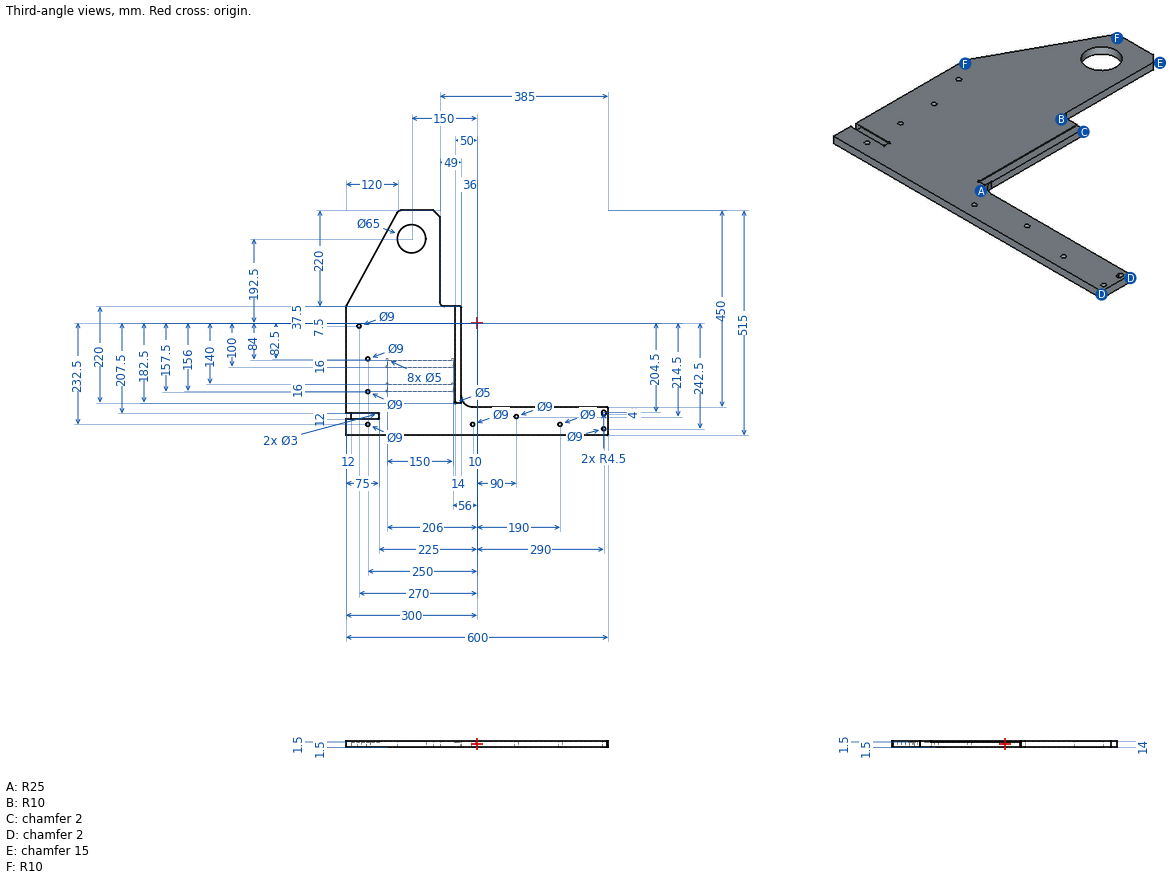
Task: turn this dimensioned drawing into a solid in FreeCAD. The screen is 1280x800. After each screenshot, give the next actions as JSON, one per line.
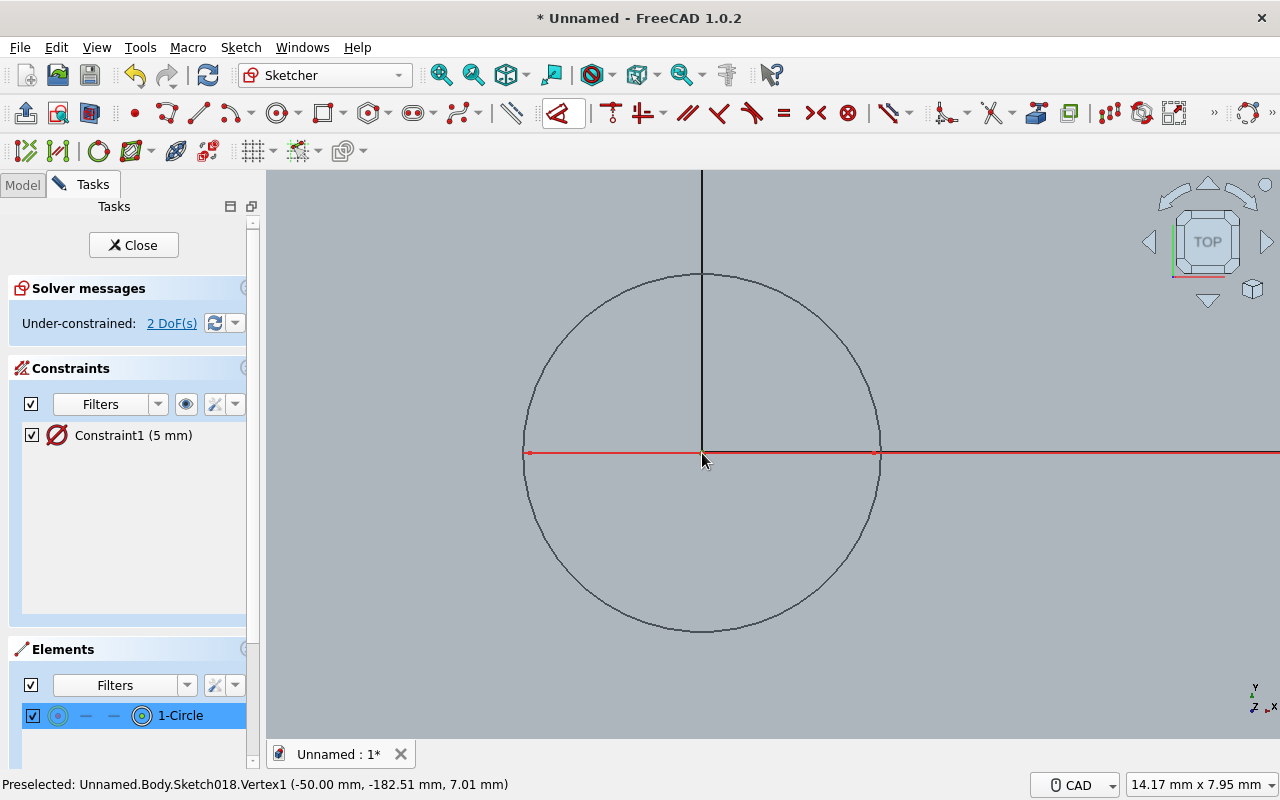
{"action": "left_click", "coordinate": [580, 114]}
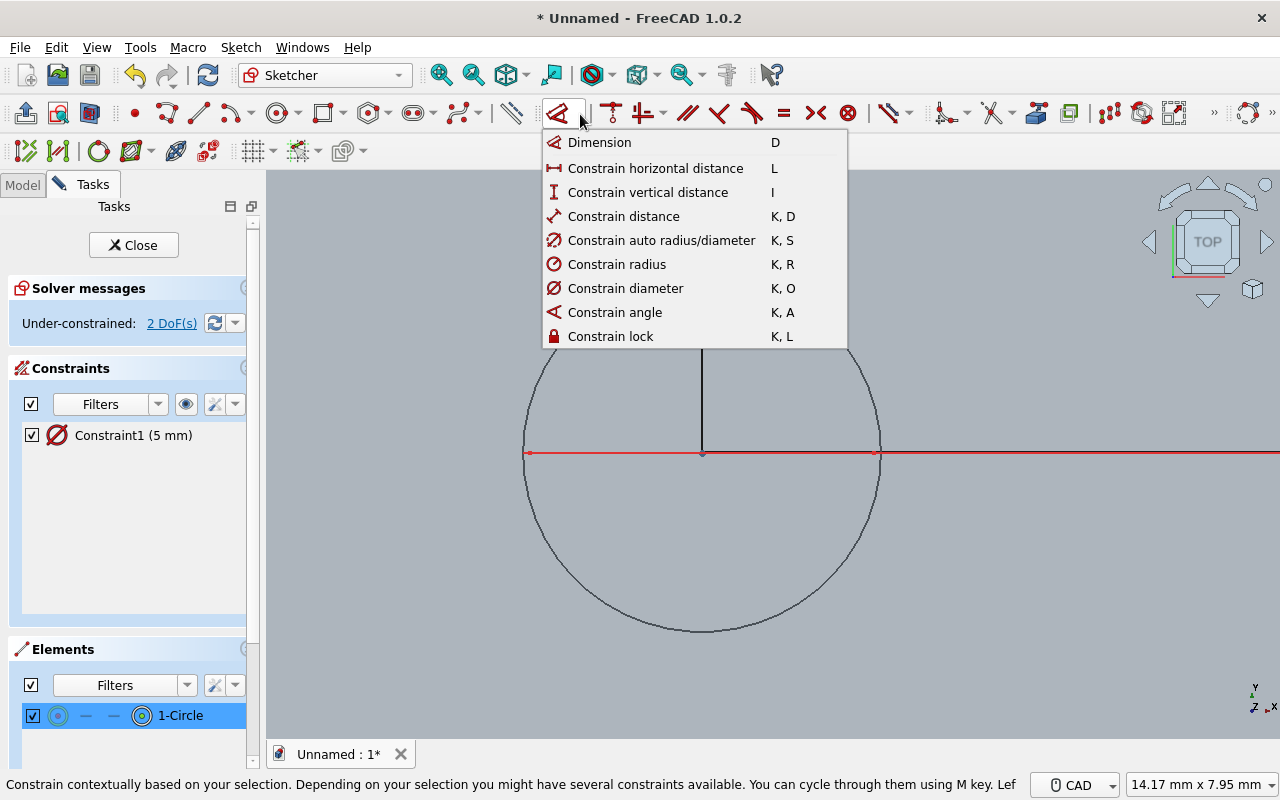
{"action": "left_click", "coordinate": [695, 168]}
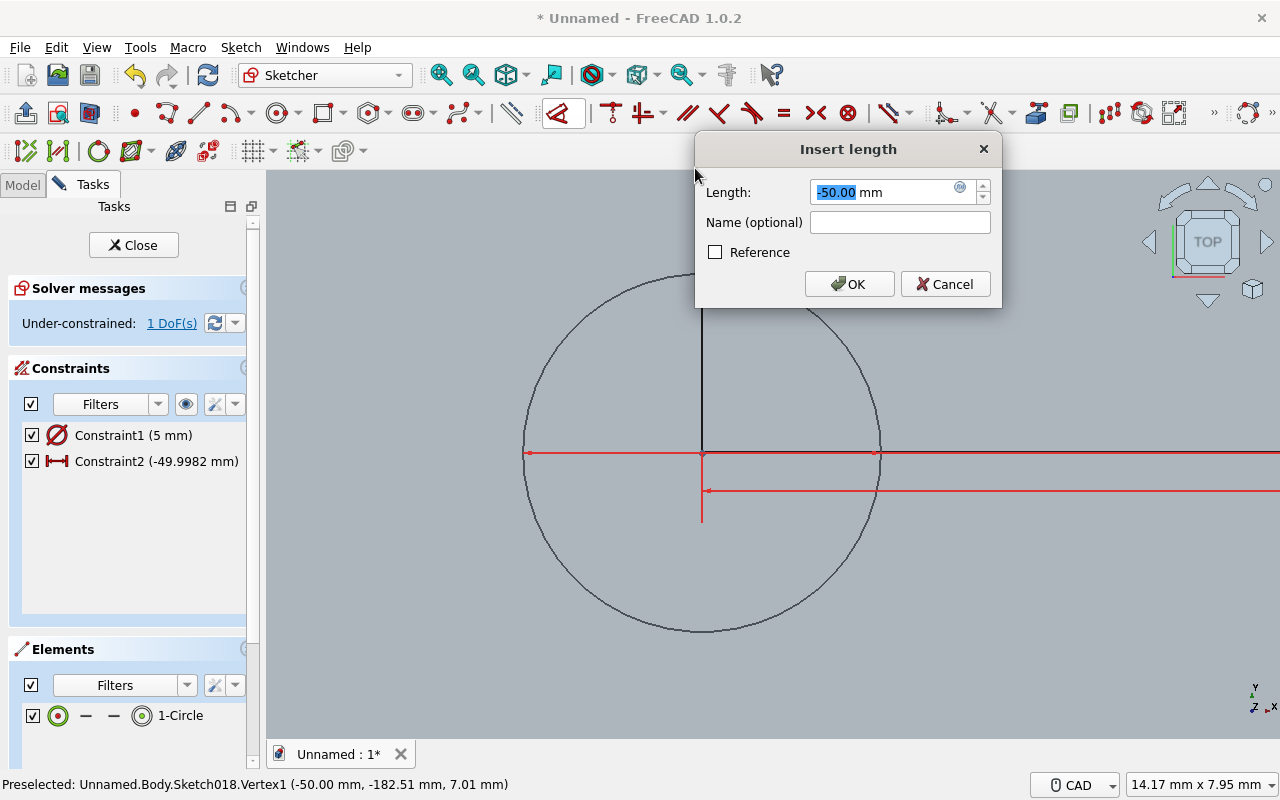
{"action": "type", "text": "-50"}
{"action": "key", "text": "Return"}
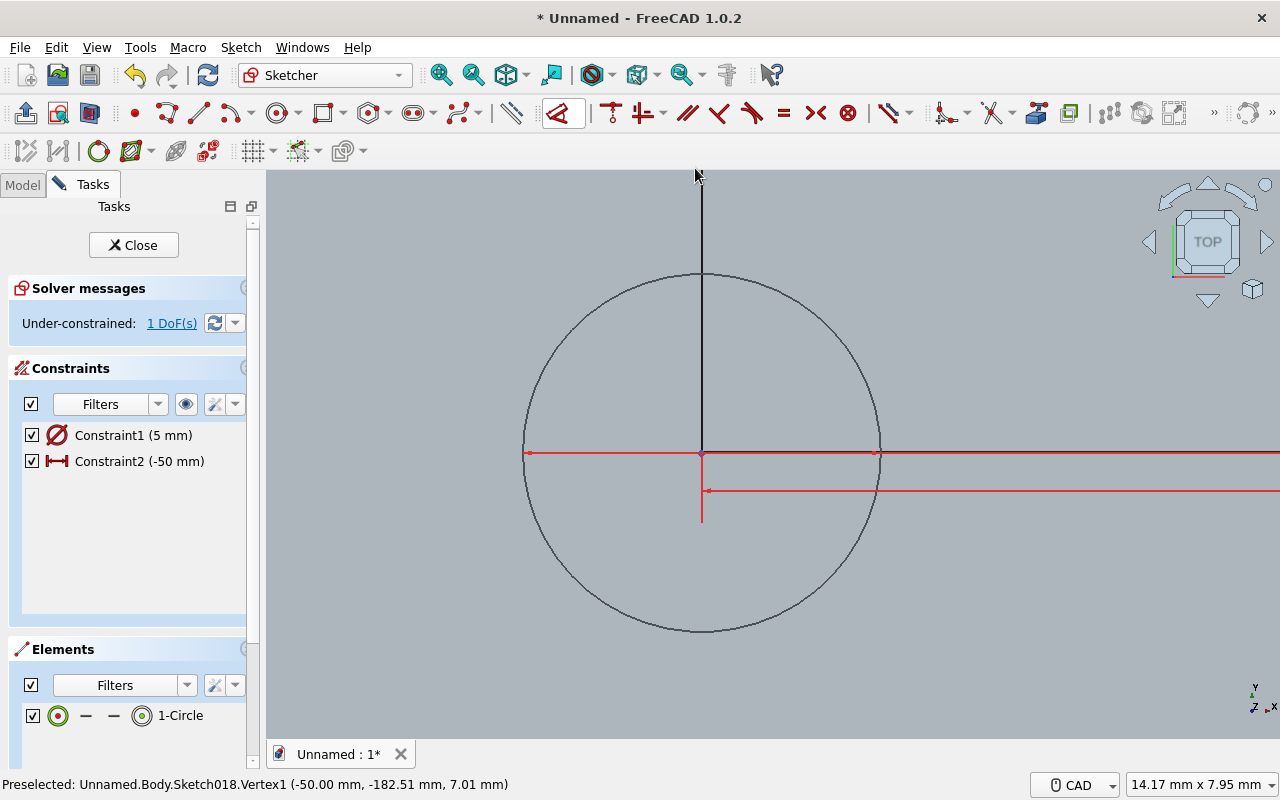
{"action": "left_click", "coordinate": [702, 453]}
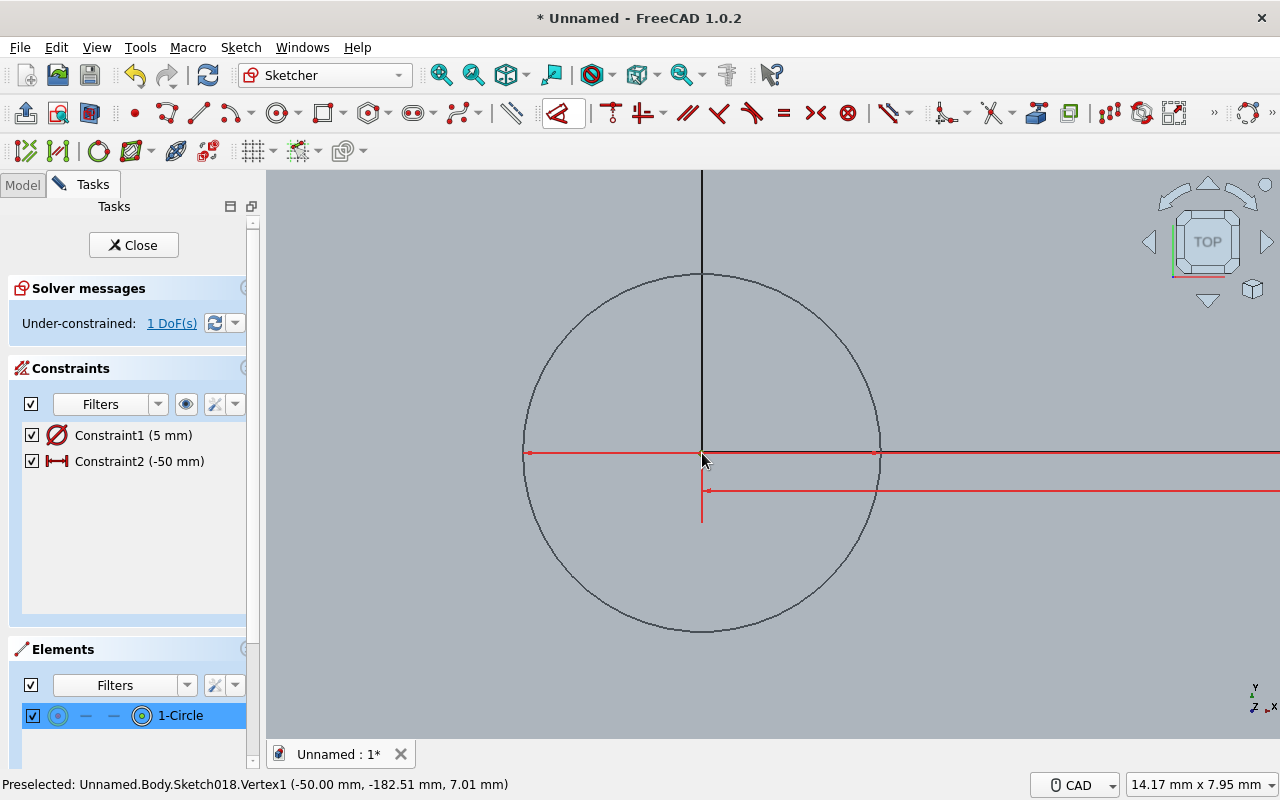
{"action": "left_click", "coordinate": [580, 114]}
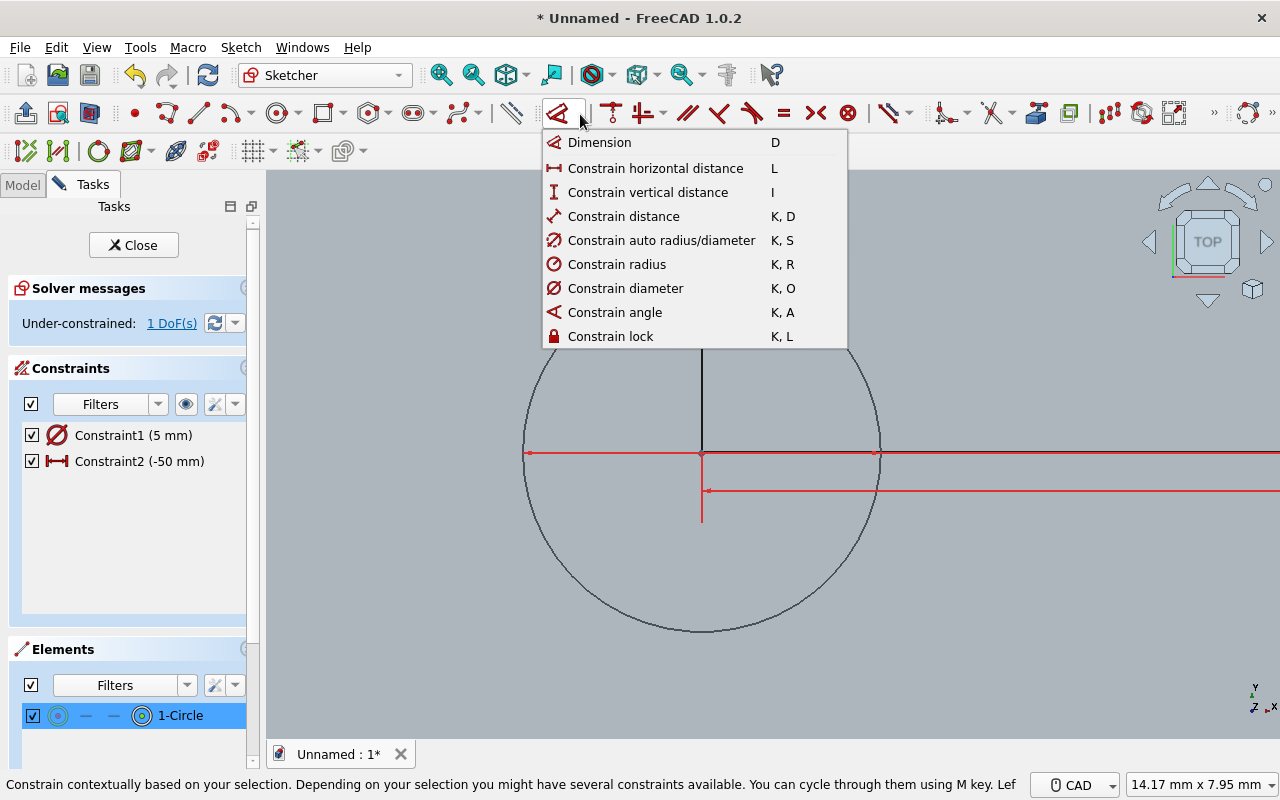
{"action": "left_click", "coordinate": [695, 192]}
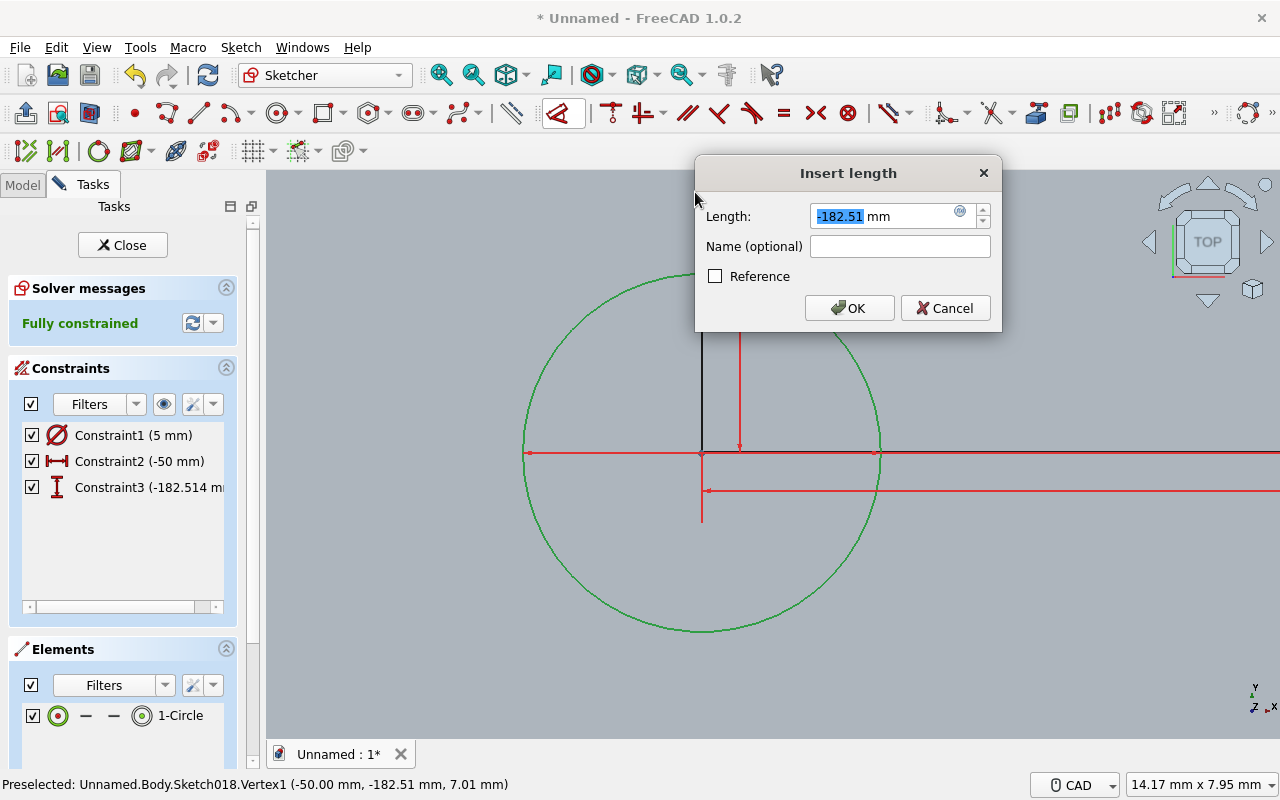
{"action": "type", "text": "-182.5"}
{"action": "key", "text": "Return"}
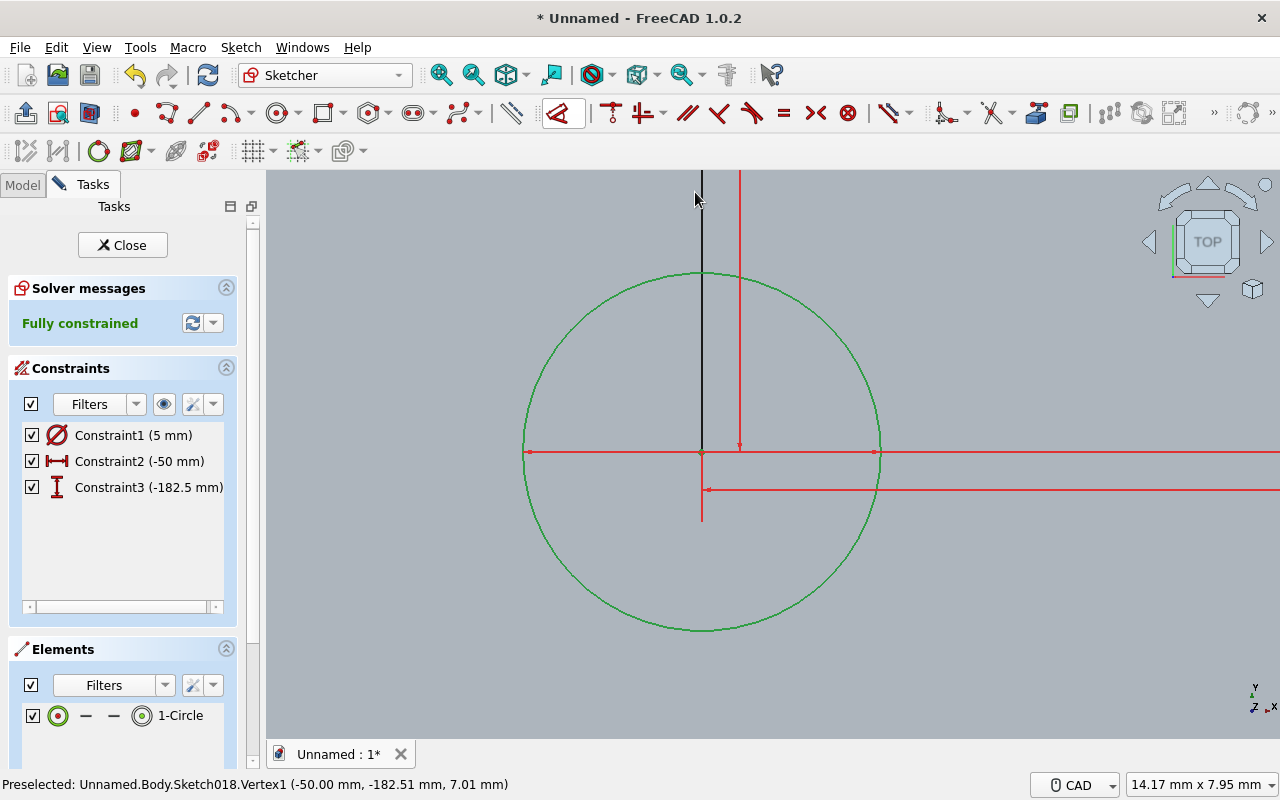
{"action": "left_click", "coordinate": [123, 245]}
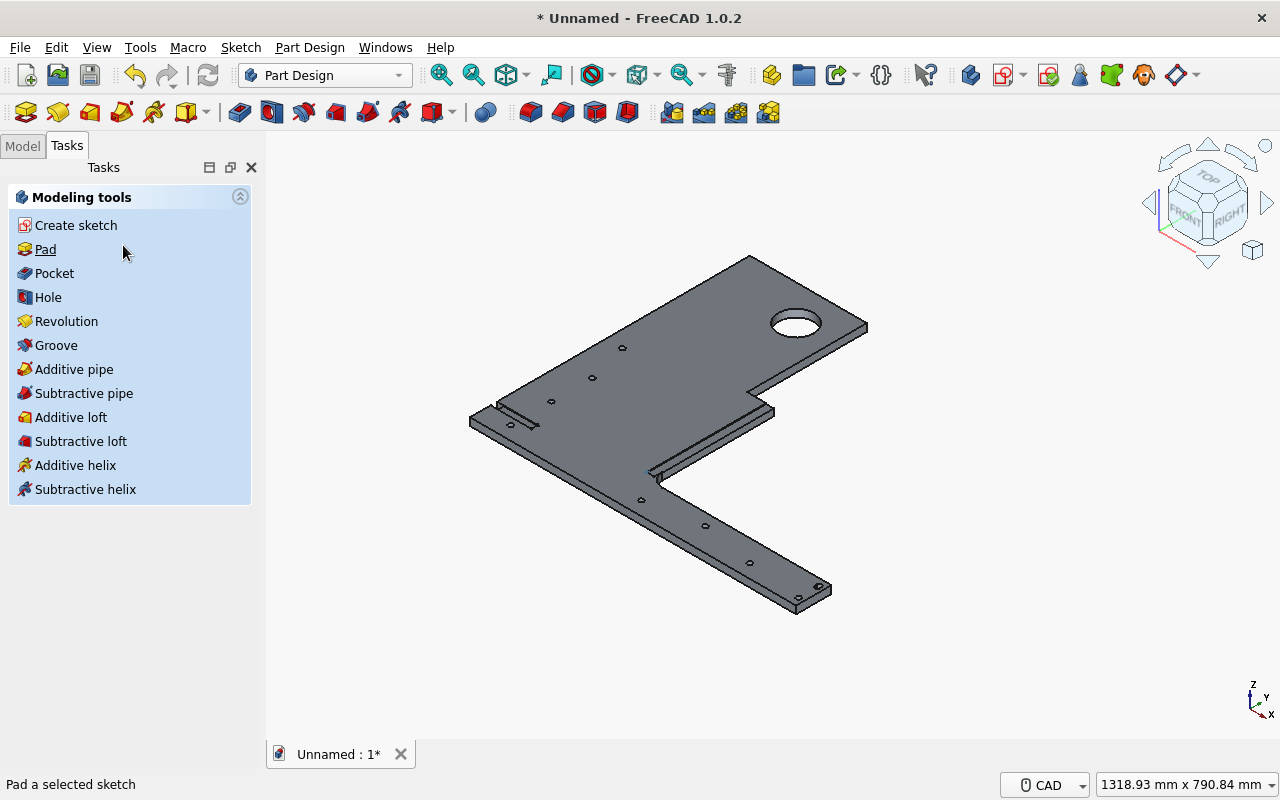
{"action": "left_click", "coordinate": [240, 112]}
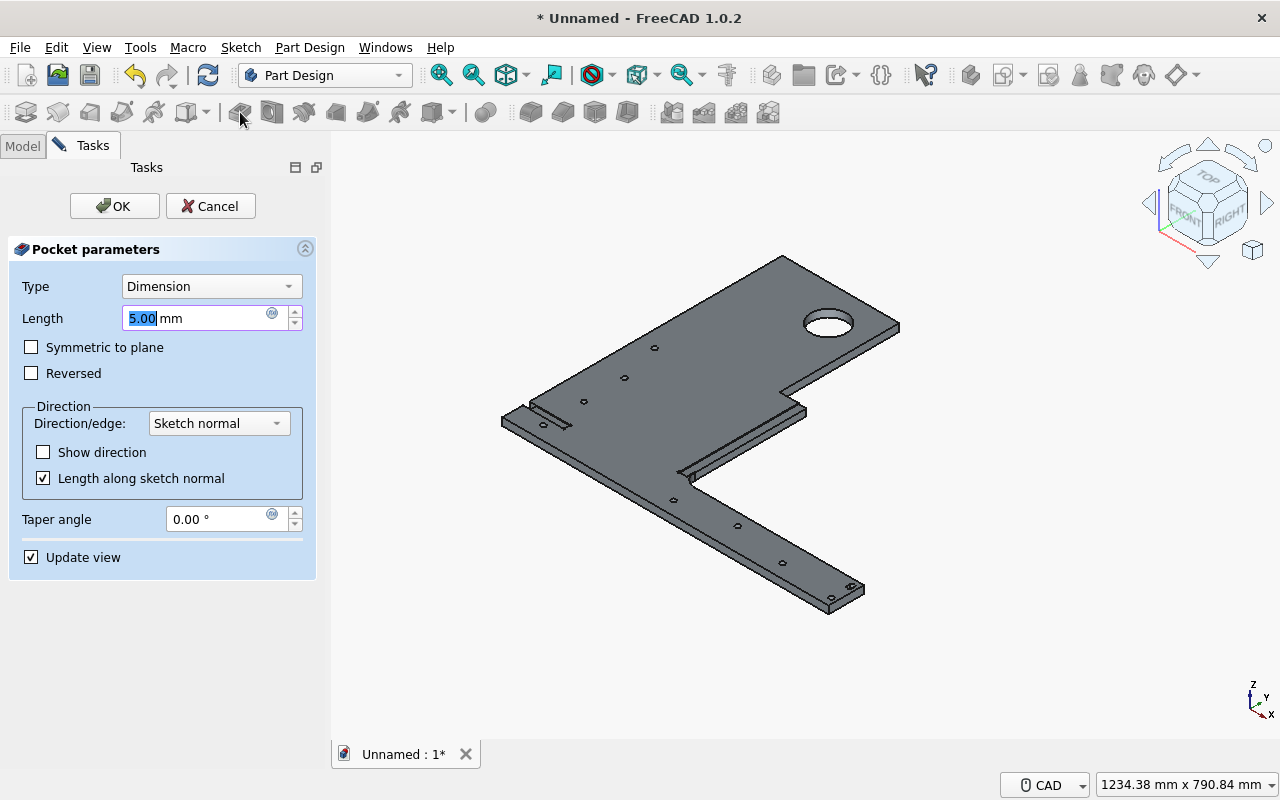
{"action": "type", "text": "1.5"}
{"action": "key", "text": "Tab"}